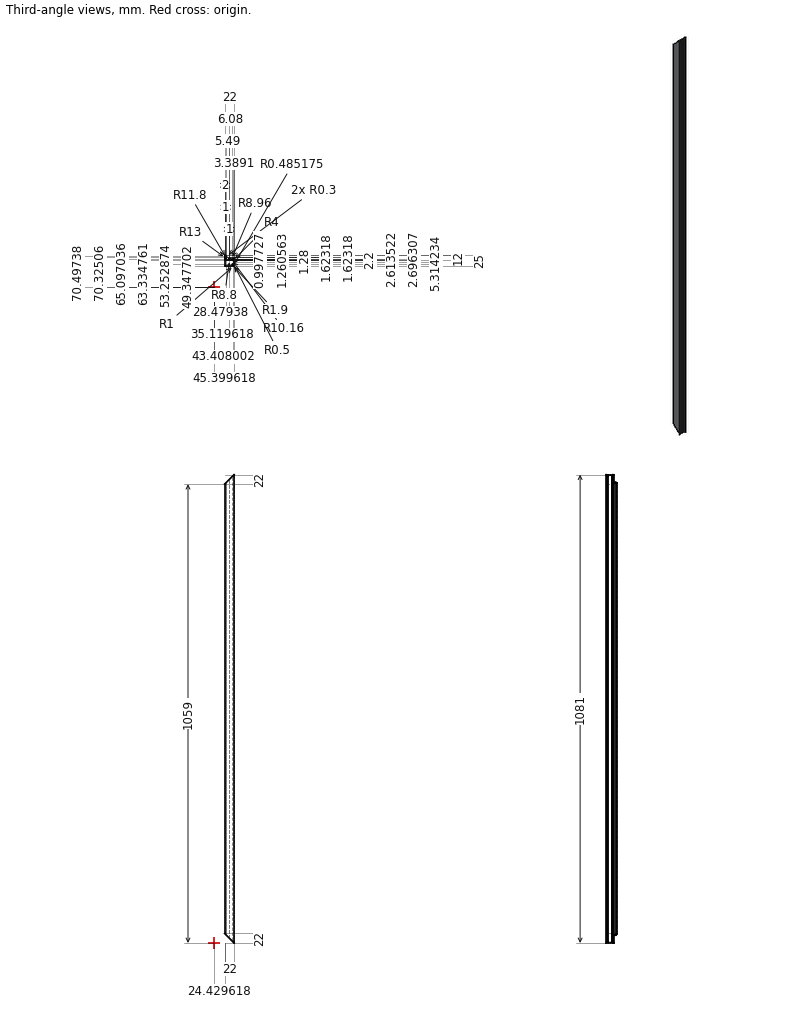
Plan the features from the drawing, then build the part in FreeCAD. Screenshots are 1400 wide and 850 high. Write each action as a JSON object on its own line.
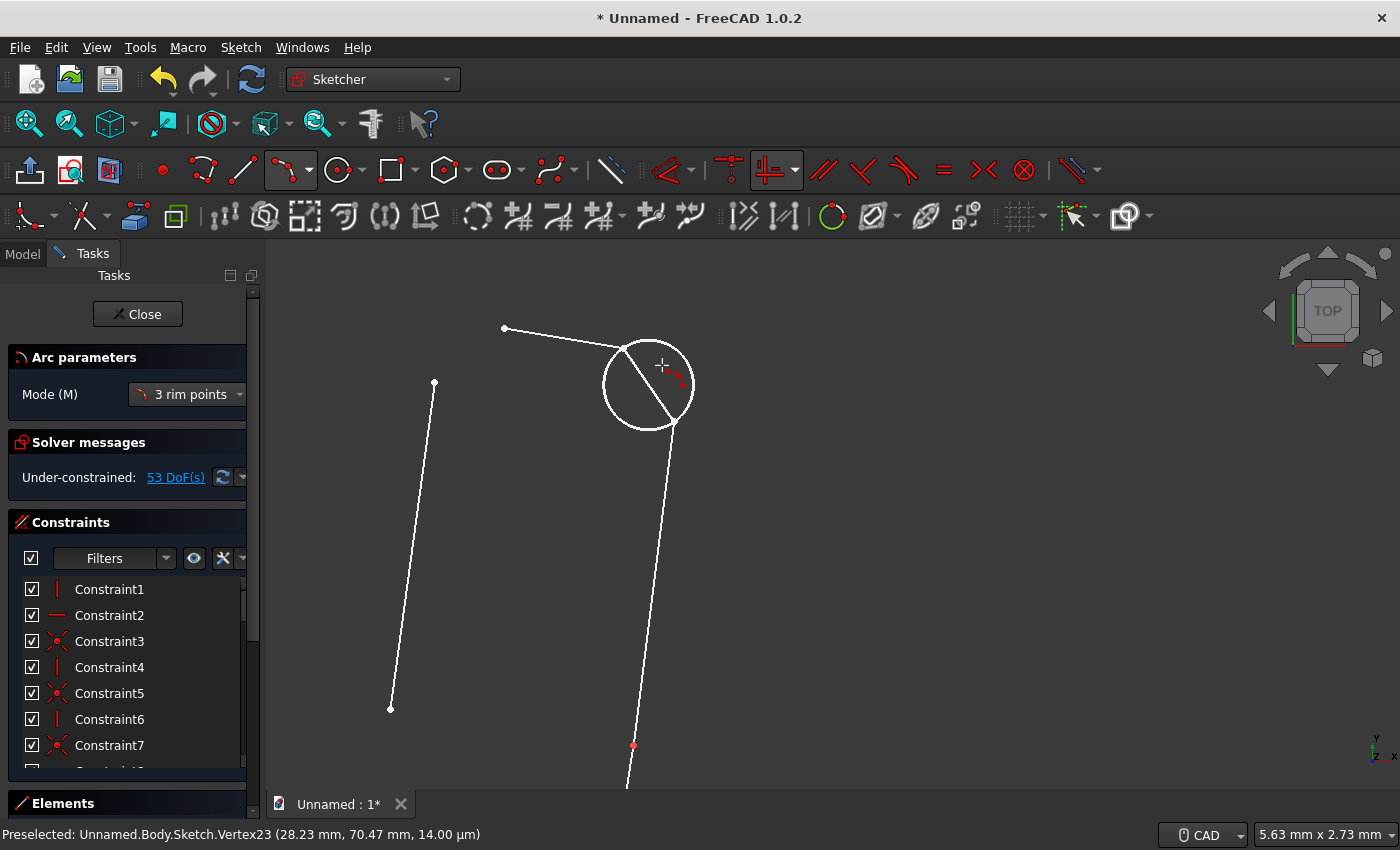
{"action": "left_click", "coordinate": [662, 365]}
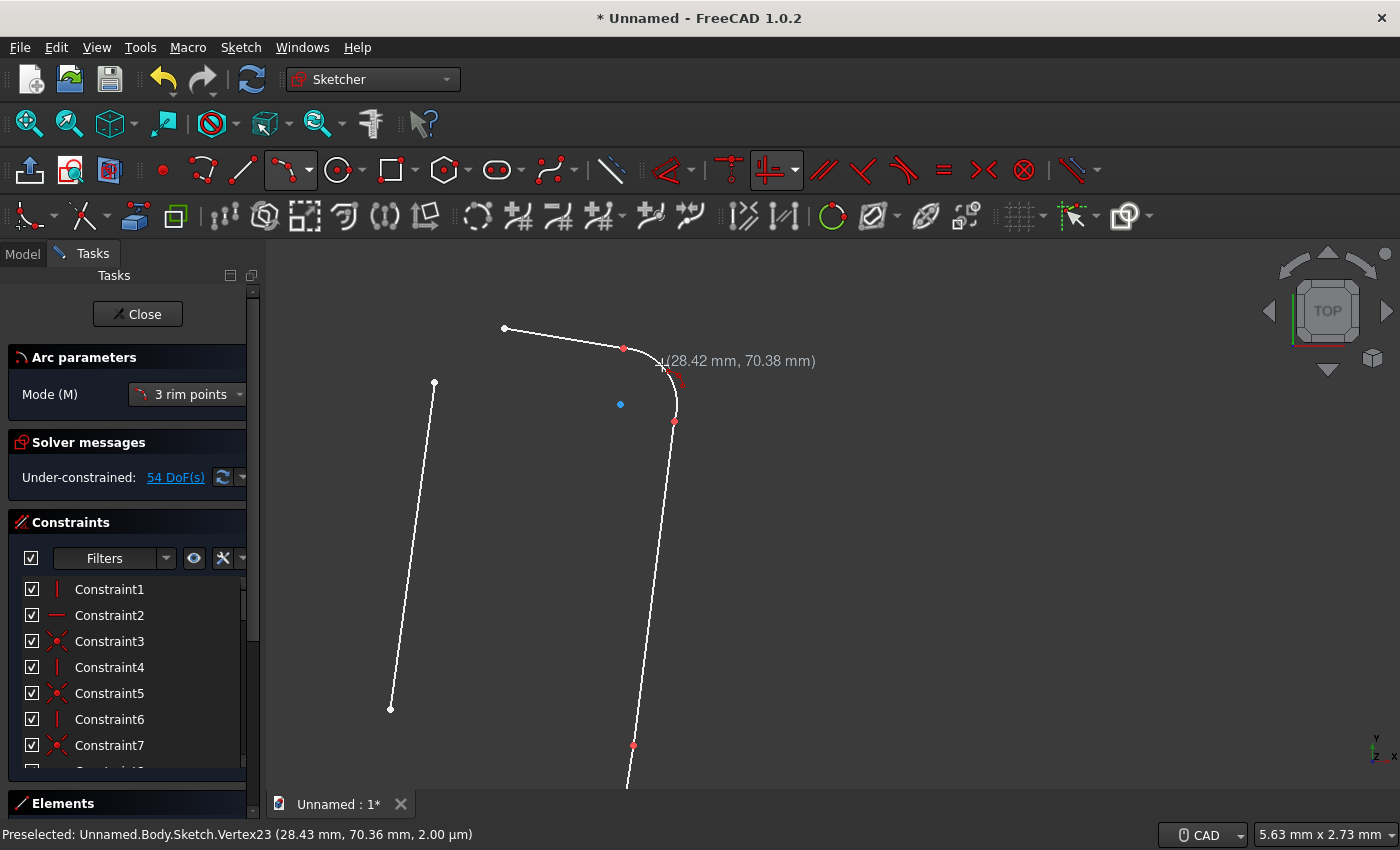
{"action": "scroll", "coordinate": [660, 370], "scroll_direction": "down", "scroll_amount": 13}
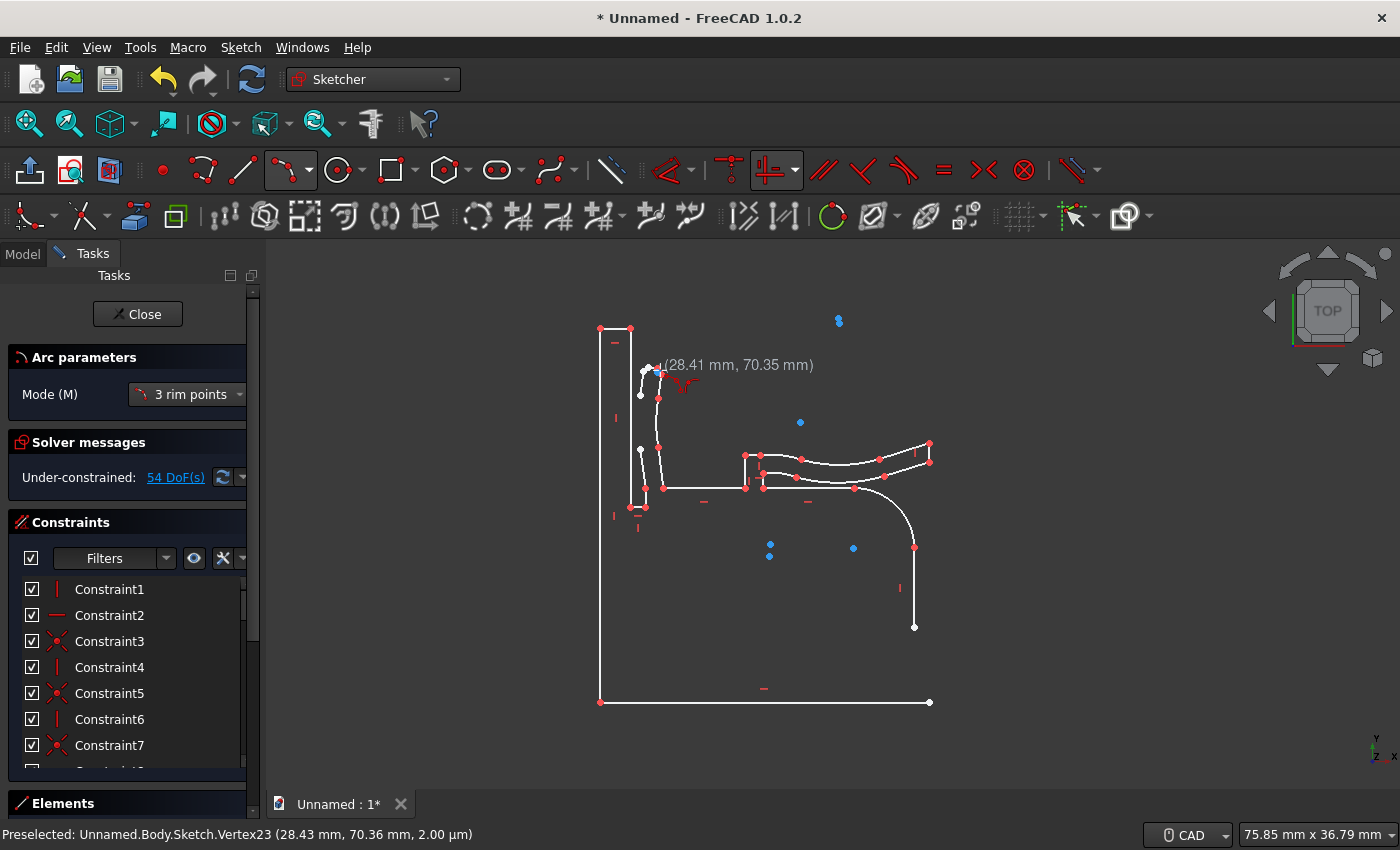
{"action": "scroll", "coordinate": [649, 367], "scroll_direction": "up", "scroll_amount": 7}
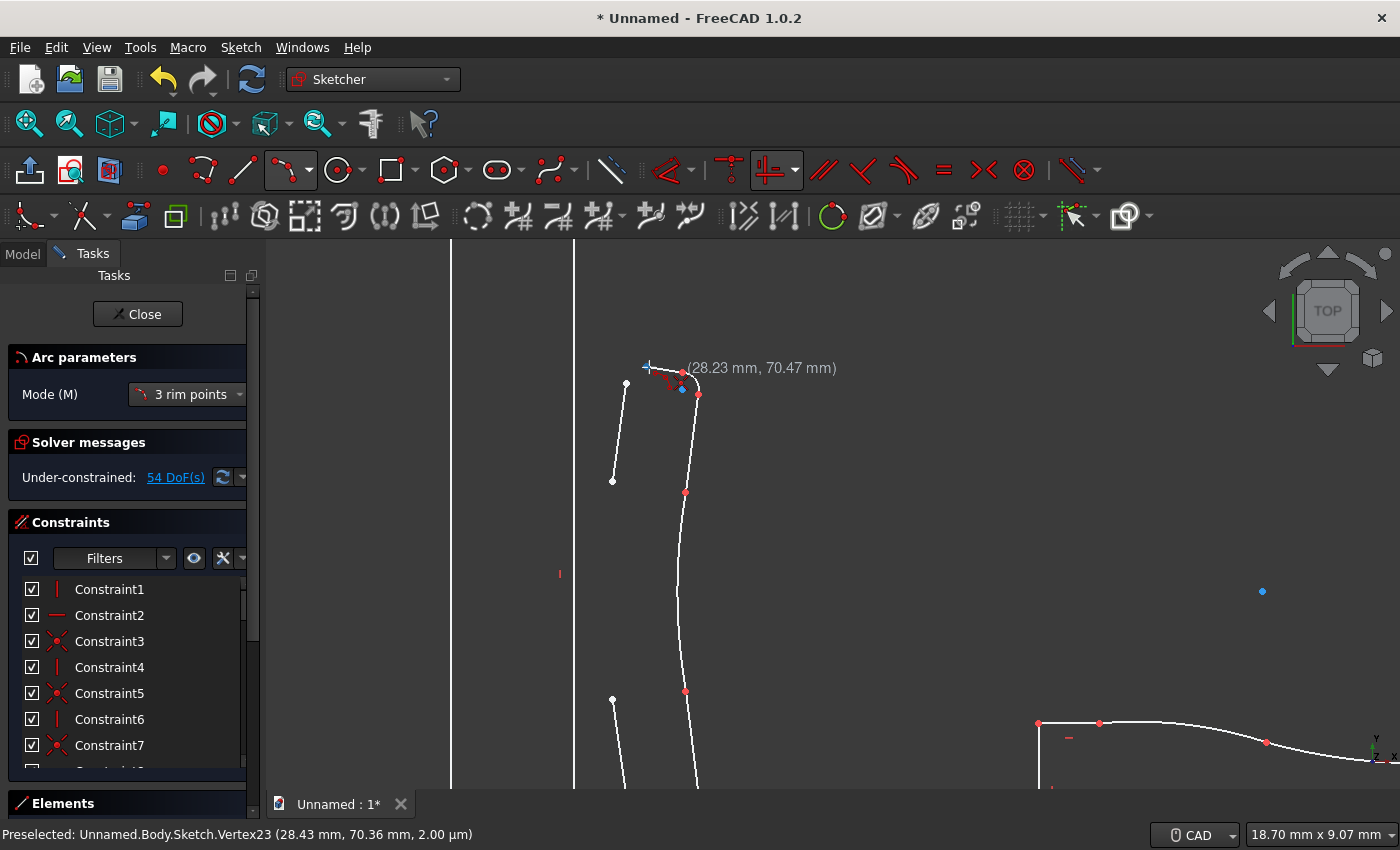
{"action": "left_click", "coordinate": [647, 367]}
{"action": "left_click", "coordinate": [626, 383]}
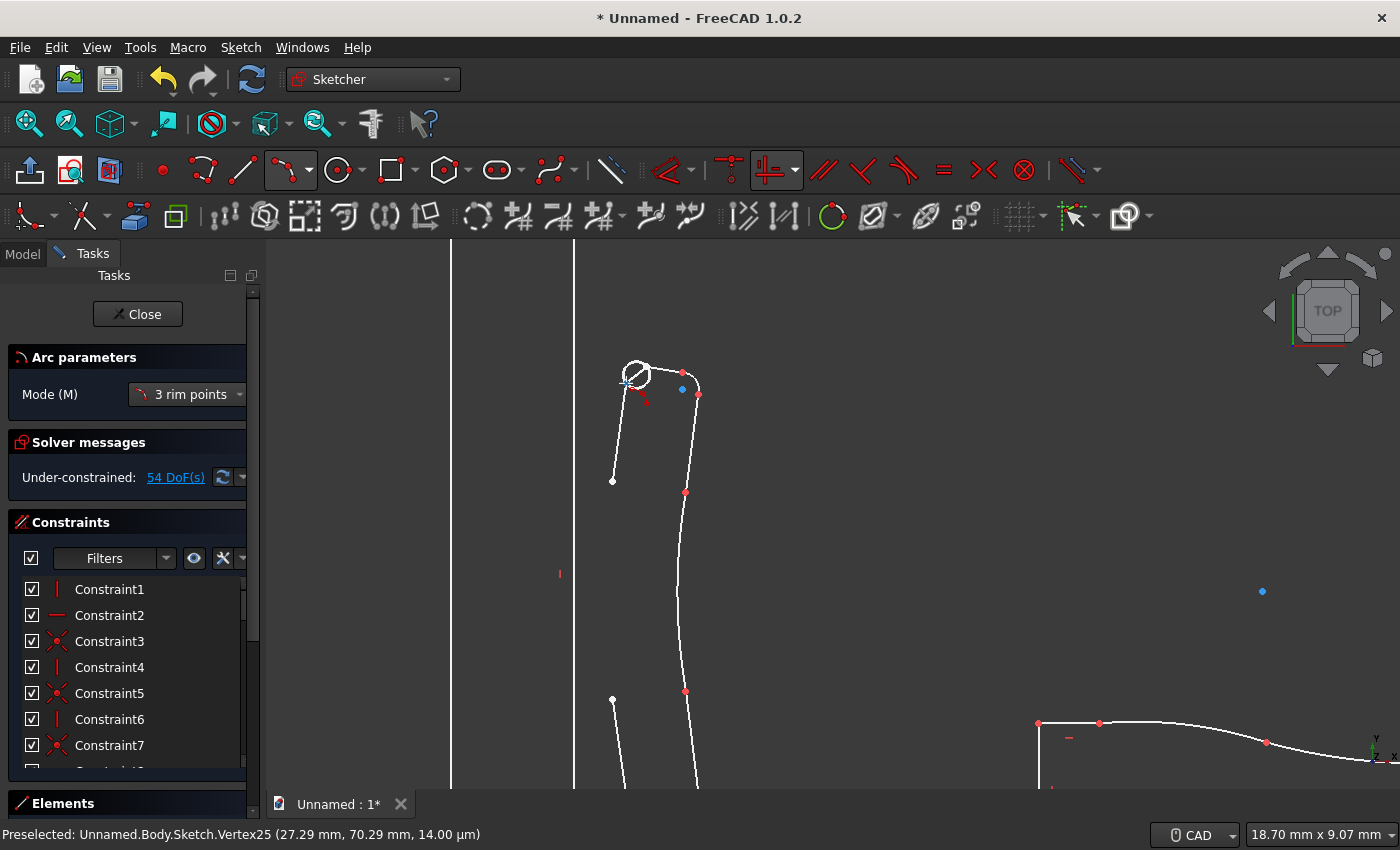
{"action": "scroll", "coordinate": [633, 369], "scroll_direction": "up", "scroll_amount": 6}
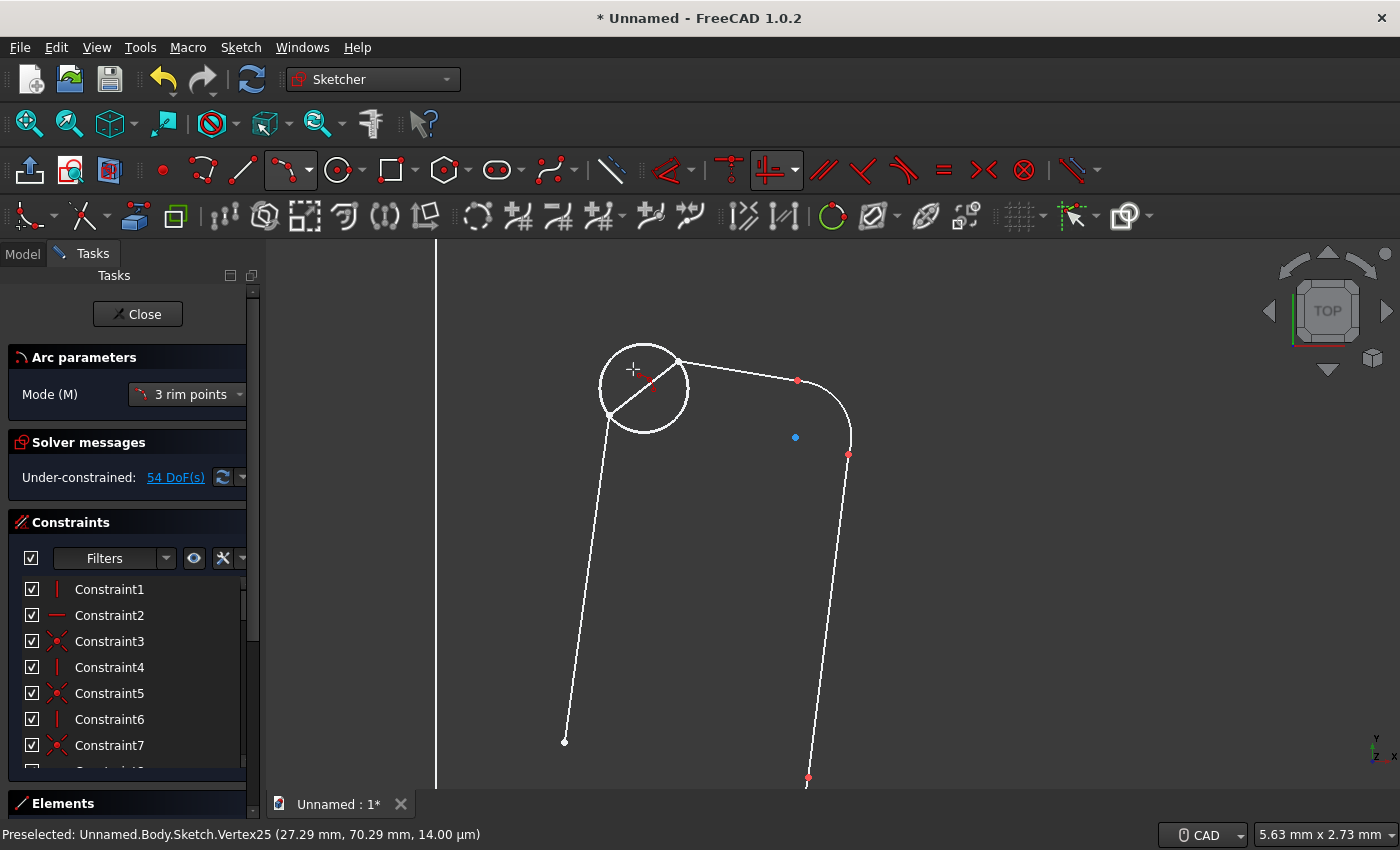
{"action": "left_click", "coordinate": [633, 370]}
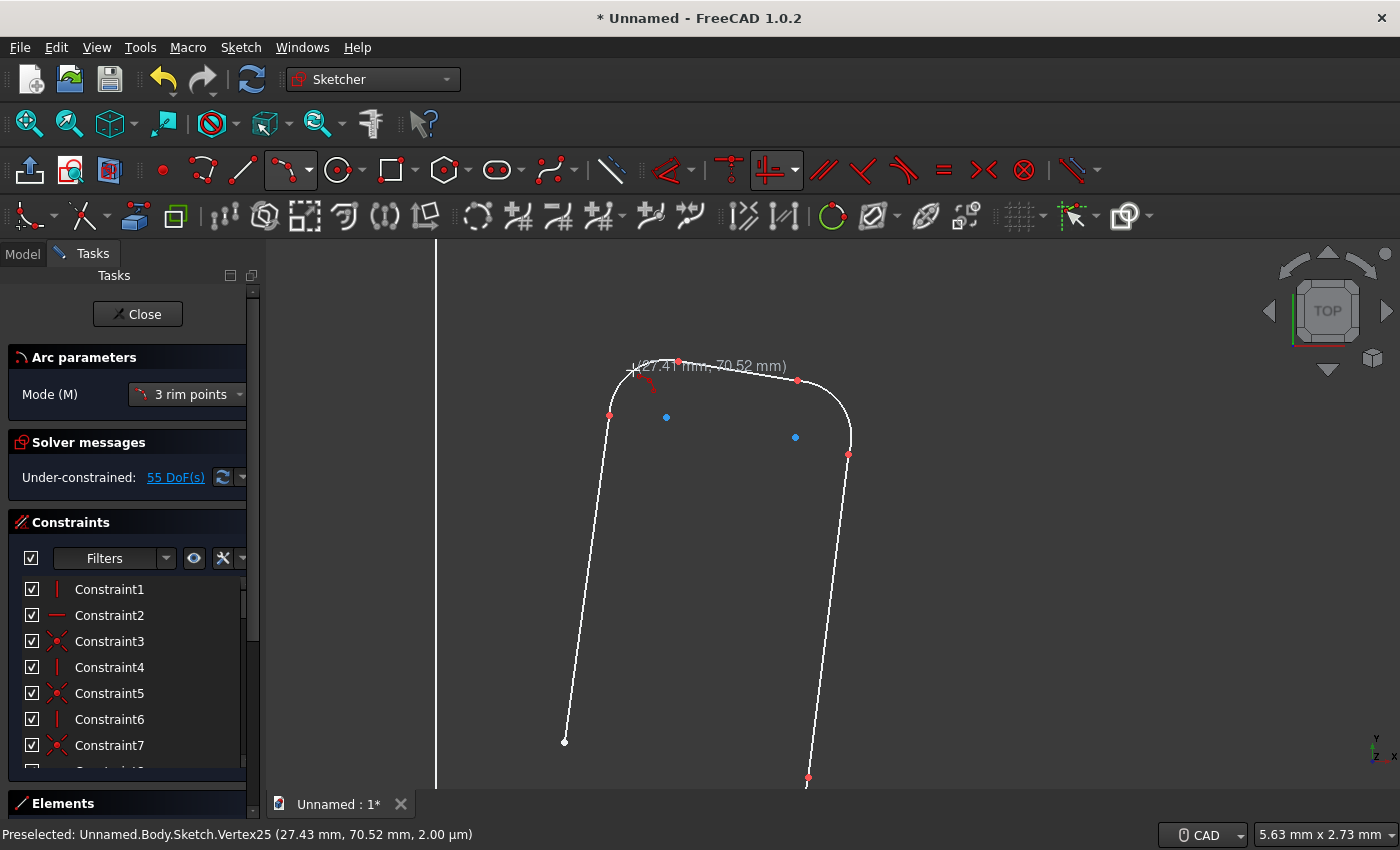
{"action": "scroll", "coordinate": [646, 367], "scroll_direction": "down", "scroll_amount": 13}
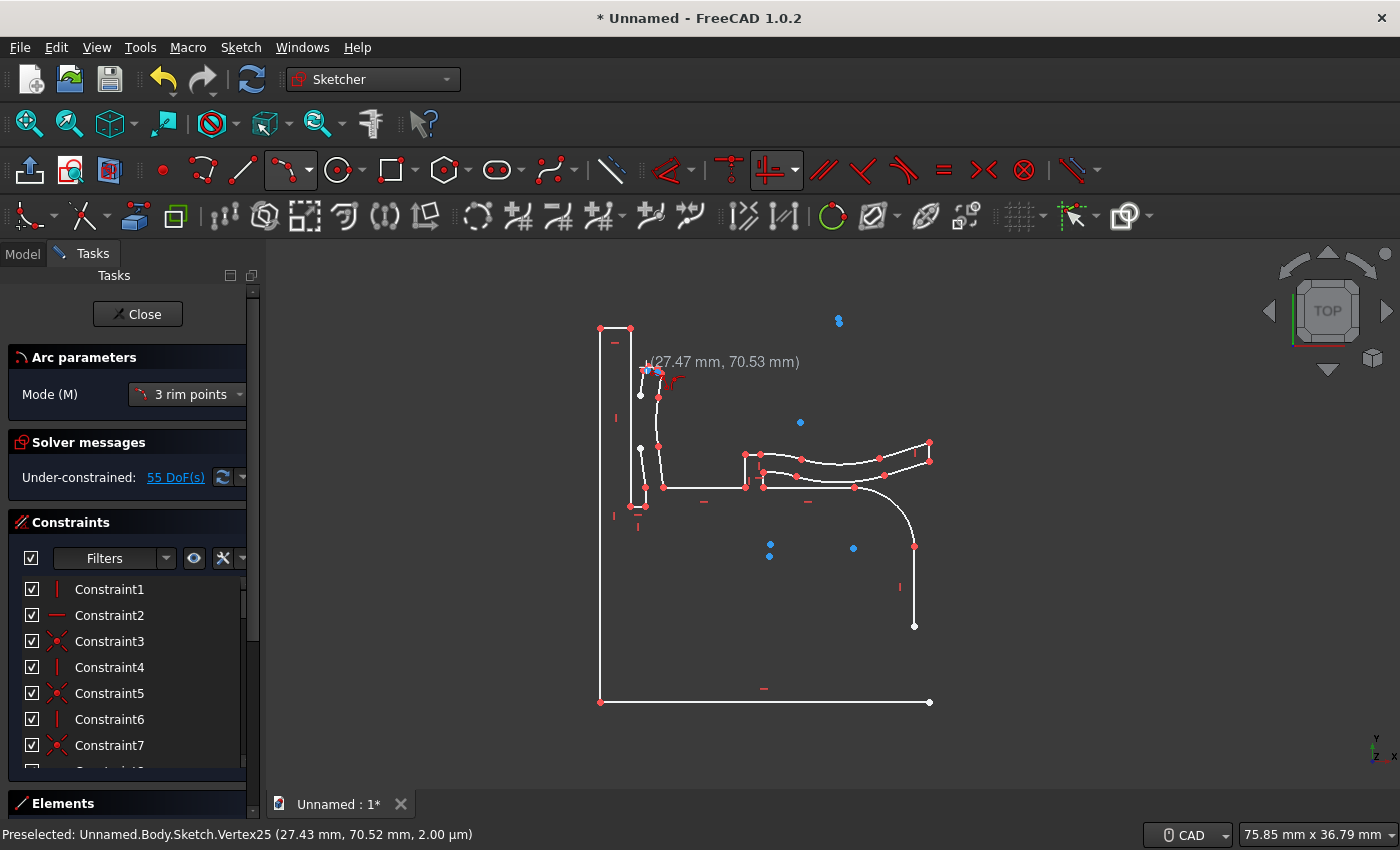
{"action": "scroll", "coordinate": [640, 395], "scroll_direction": "up", "scroll_amount": 3}